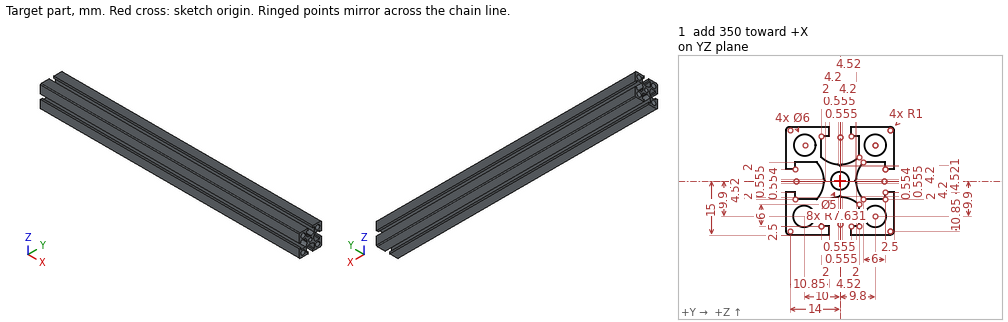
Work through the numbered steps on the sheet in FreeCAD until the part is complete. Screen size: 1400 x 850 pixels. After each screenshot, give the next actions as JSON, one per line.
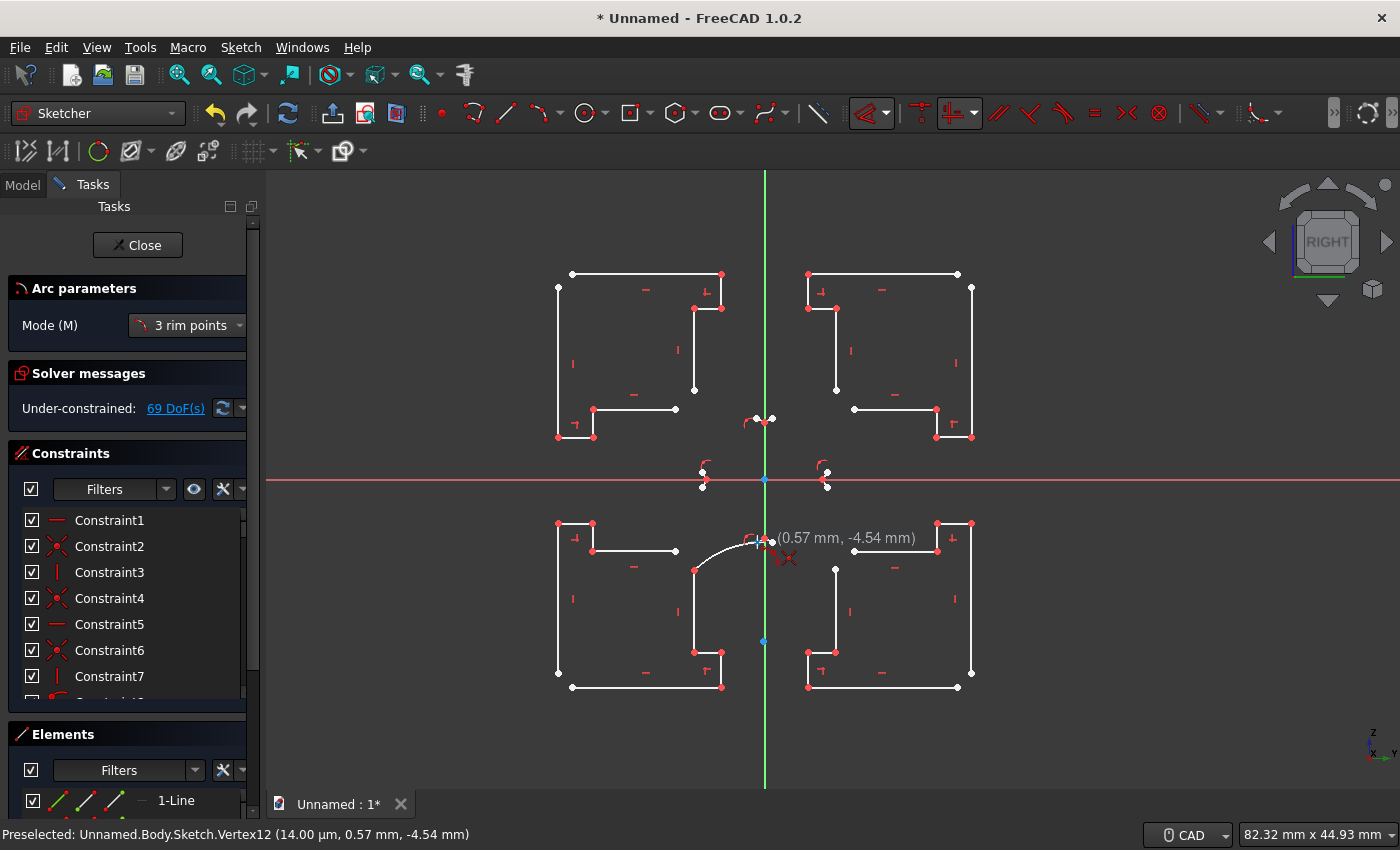
{"action": "left_click", "coordinate": [836, 570]}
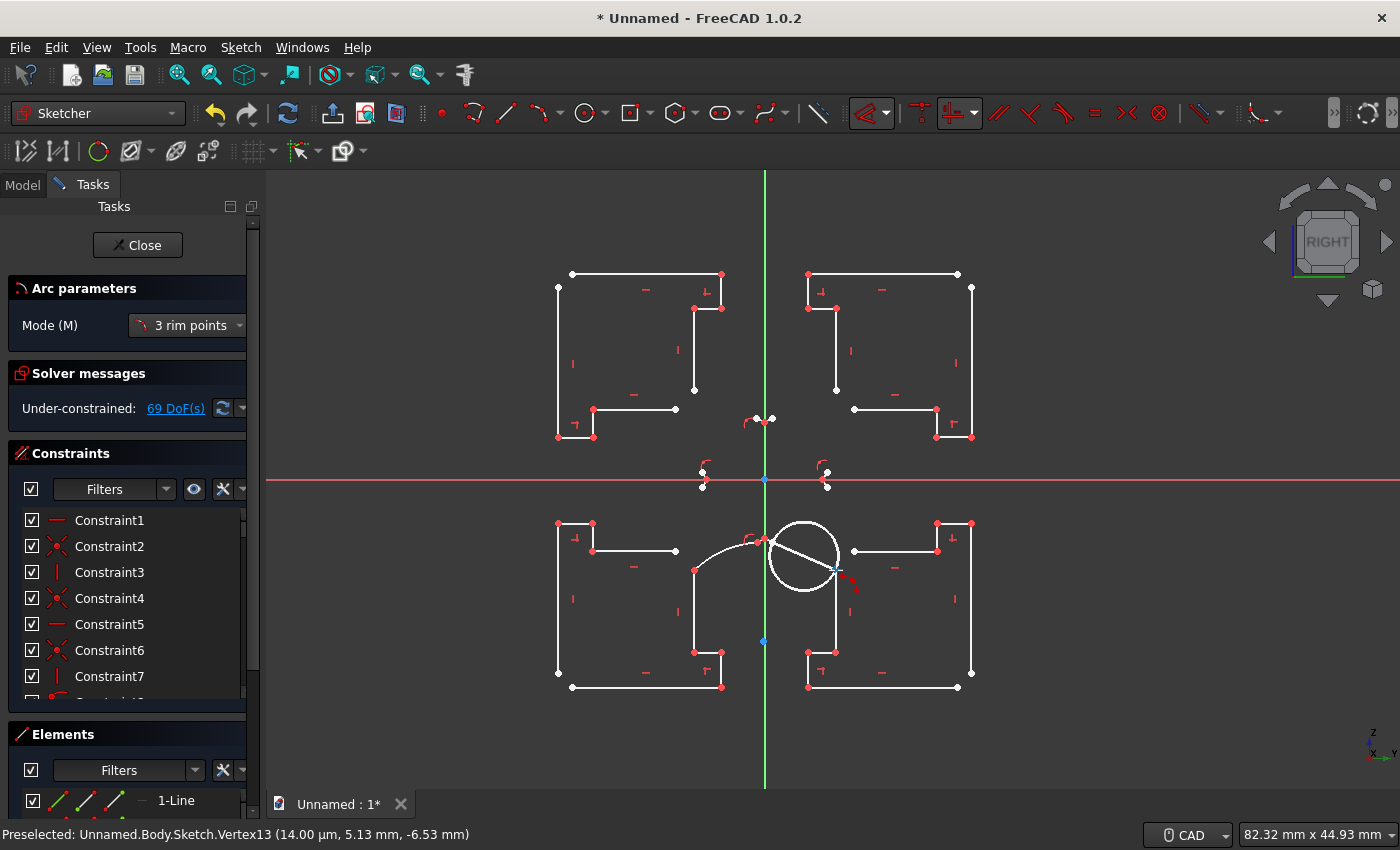
{"action": "scroll", "coordinate": [806, 550], "scroll_direction": "up", "scroll_amount": 6}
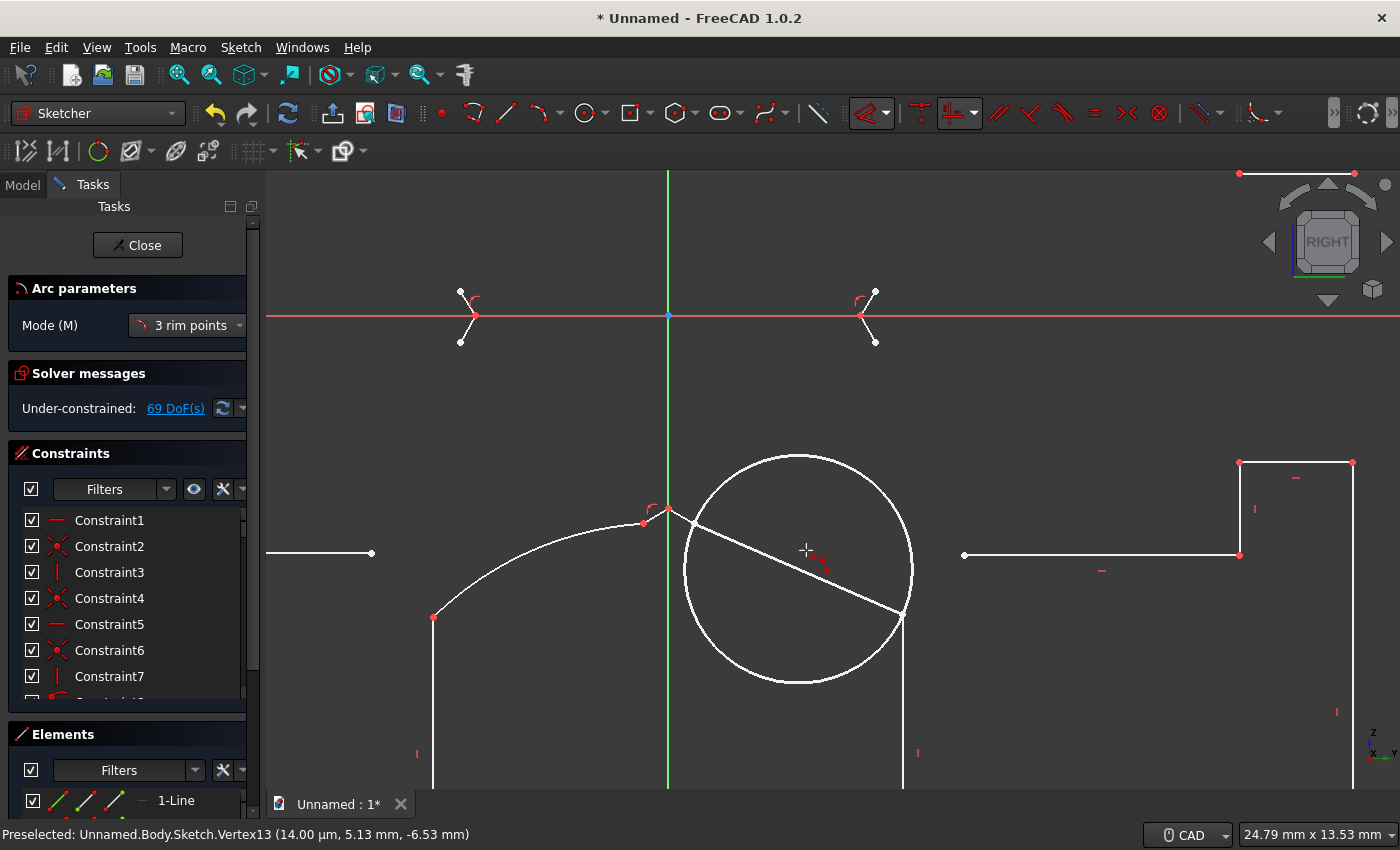
{"action": "left_click", "coordinate": [806, 550]}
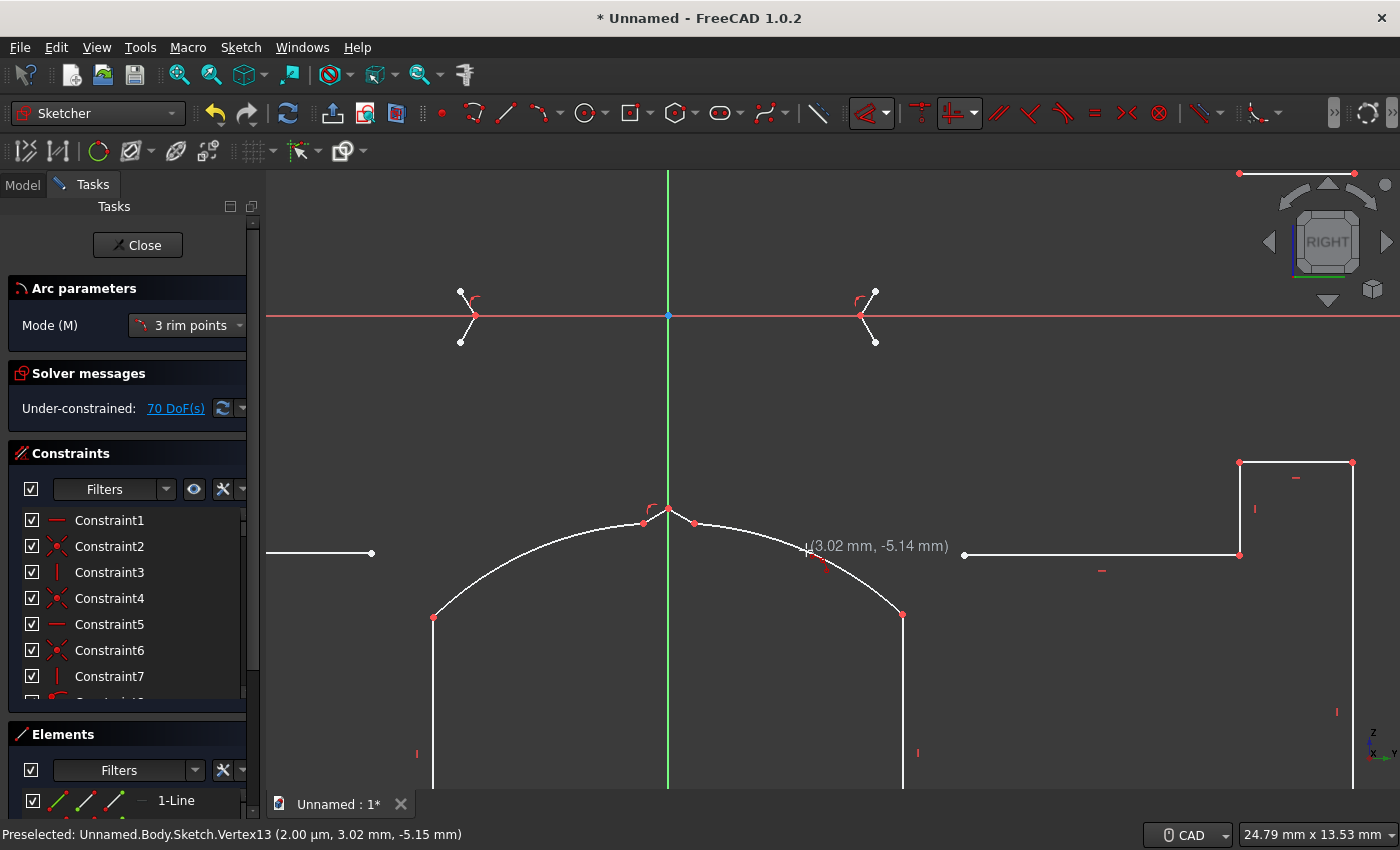
{"action": "scroll", "coordinate": [806, 550], "scroll_direction": "down", "scroll_amount": 6}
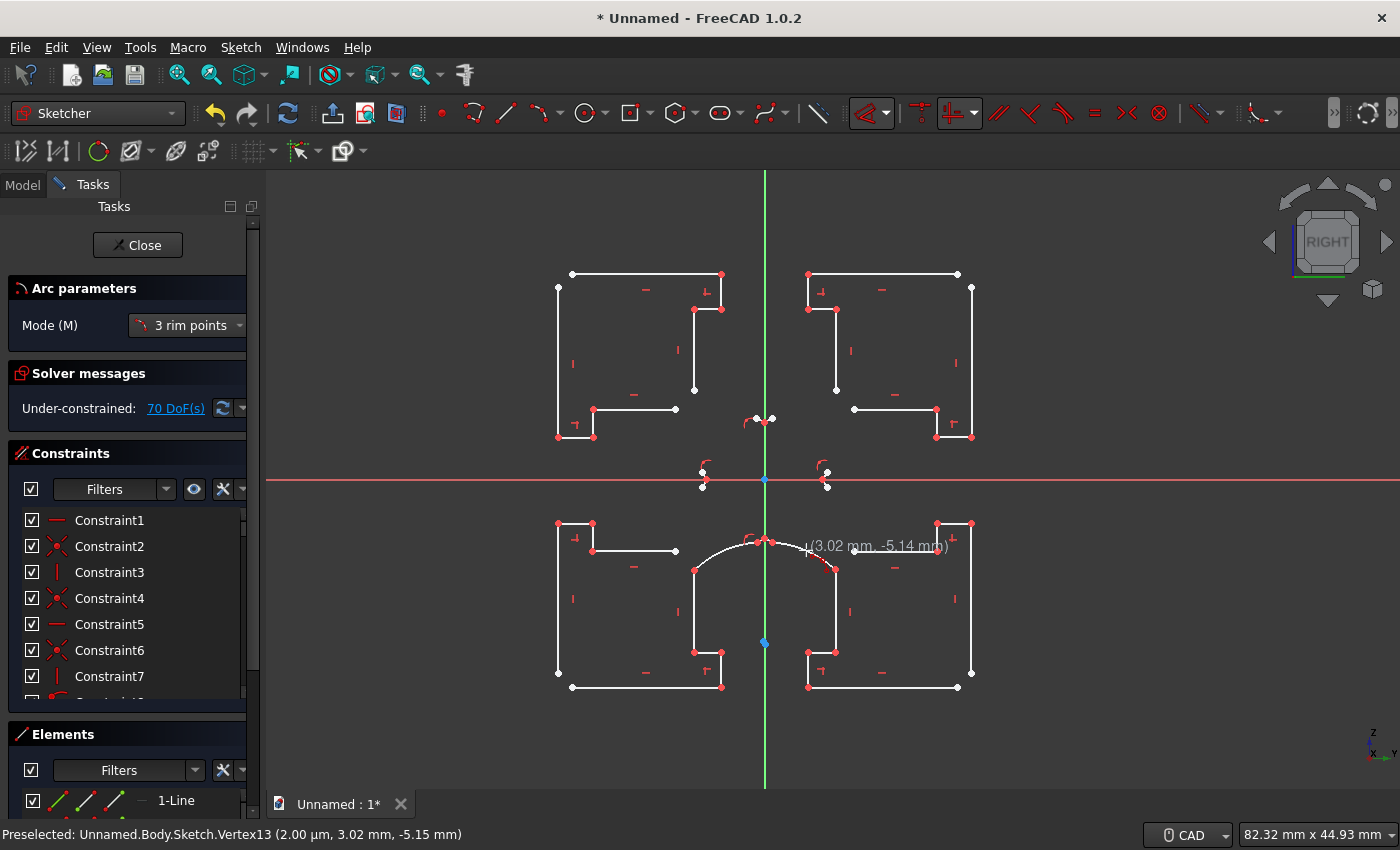
{"action": "left_click", "coordinate": [958, 688]}
{"action": "left_click", "coordinate": [971, 674]}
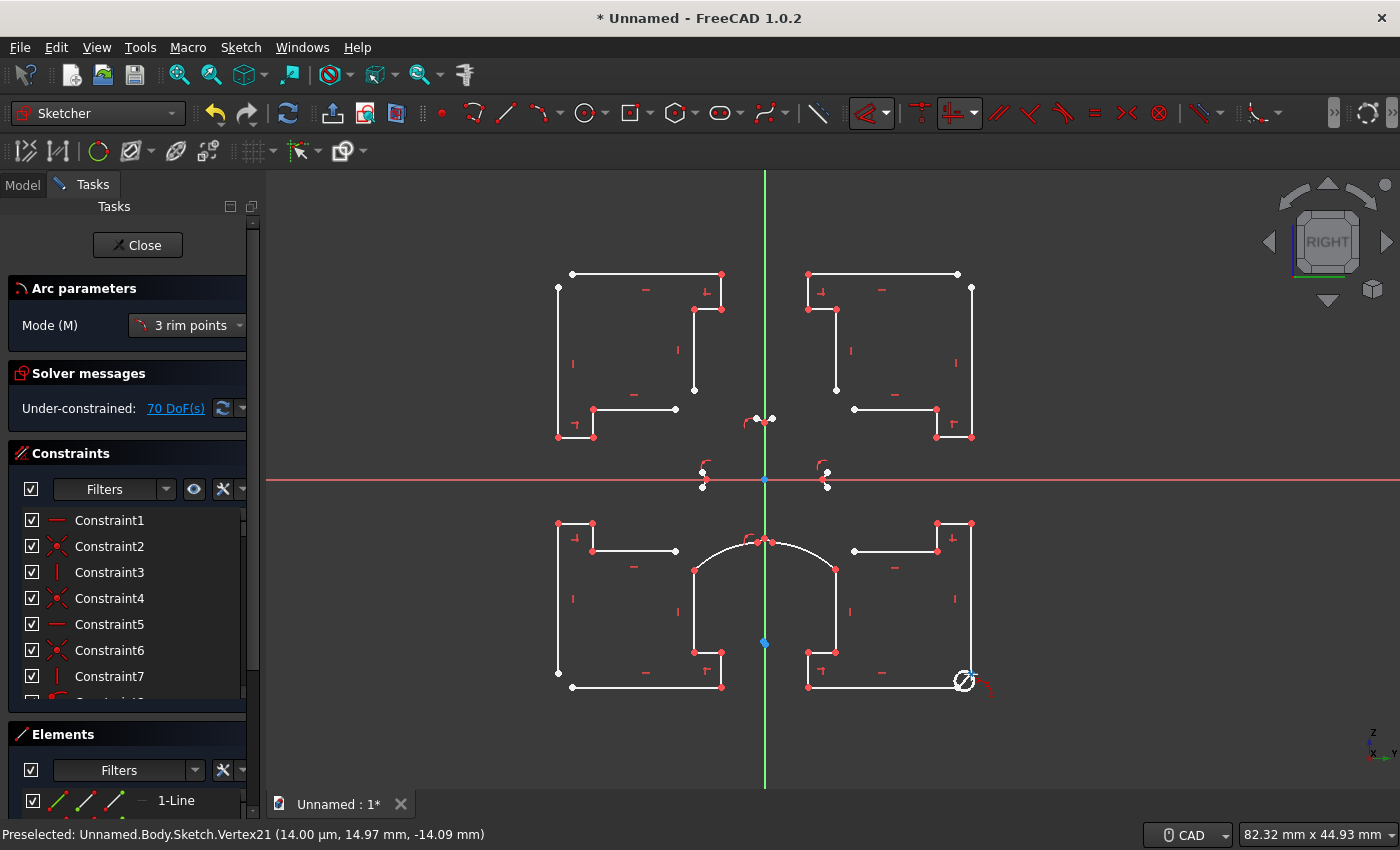
{"action": "scroll", "coordinate": [967, 683], "scroll_direction": "up", "scroll_amount": 7}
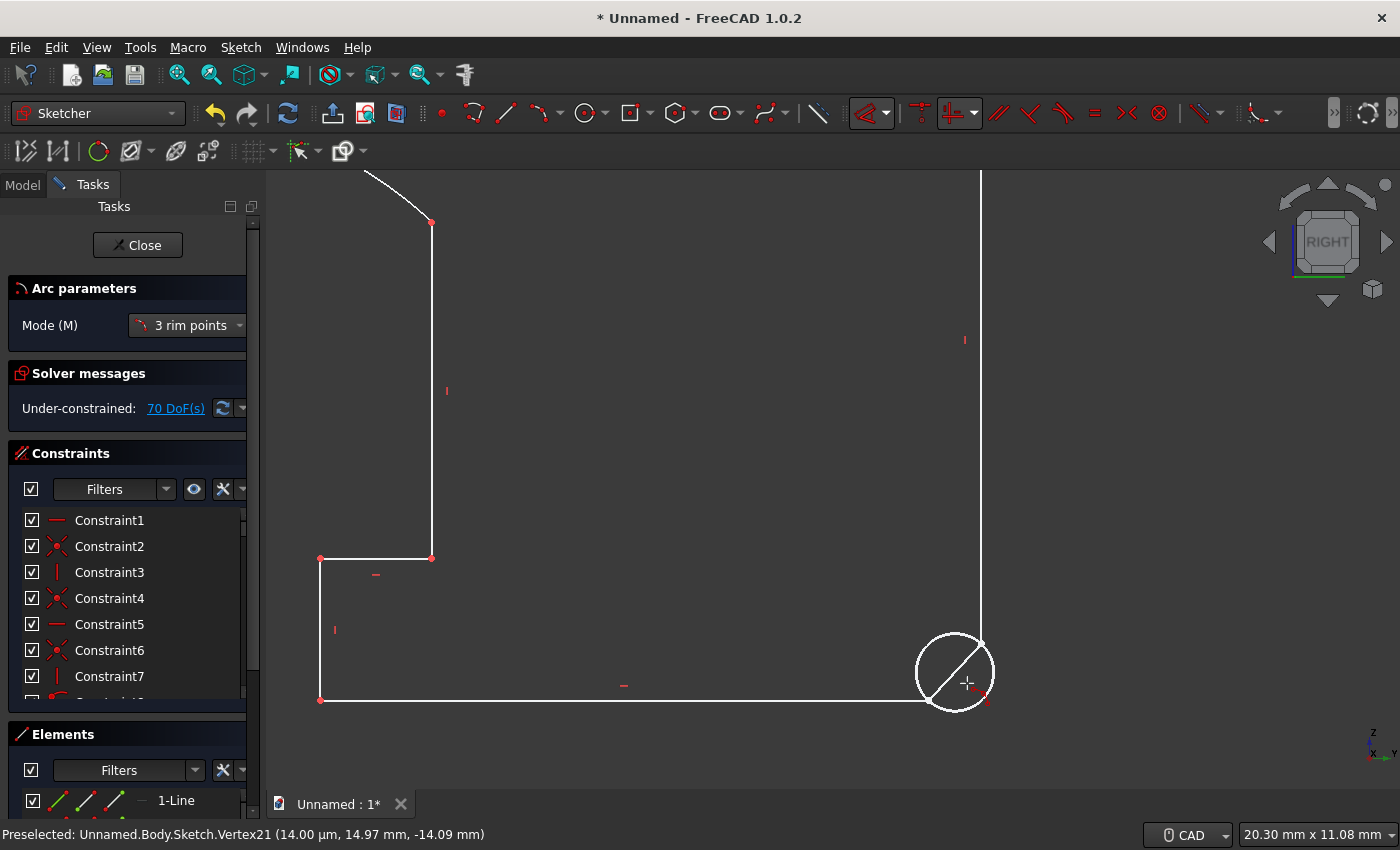
{"action": "left_click", "coordinate": [967, 679]}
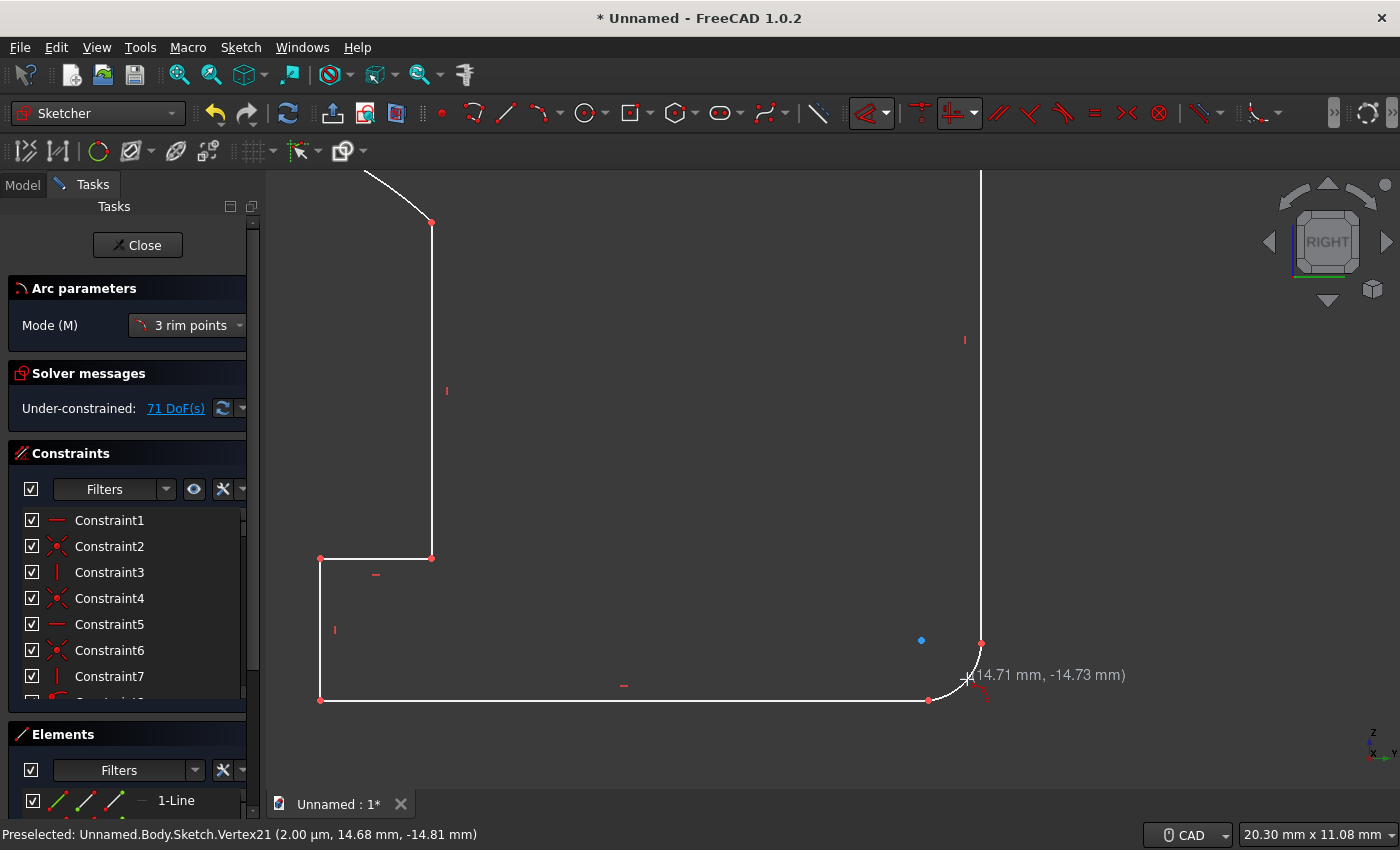
{"action": "scroll", "coordinate": [967, 683], "scroll_direction": "down", "scroll_amount": 7}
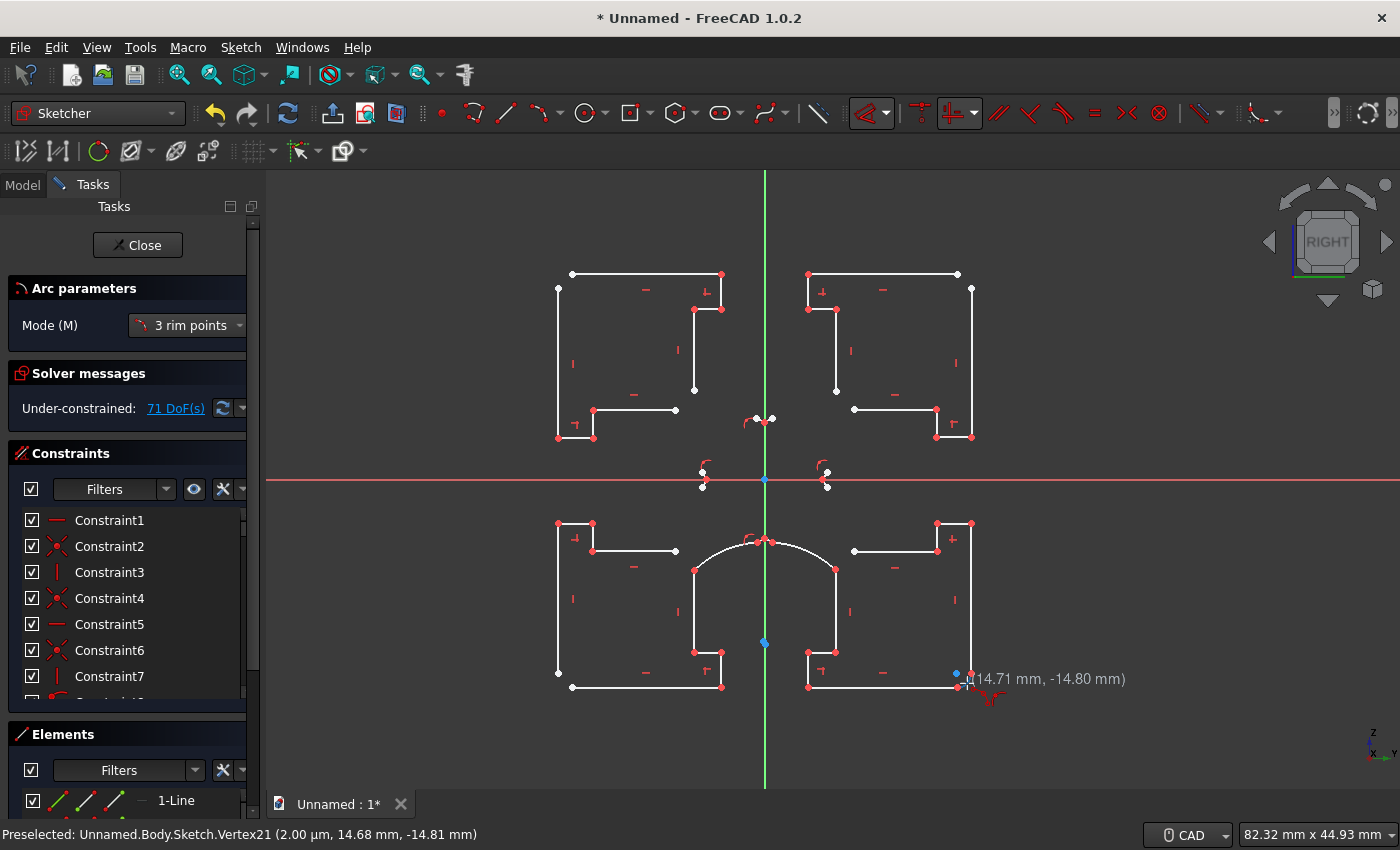
{"action": "left_click", "coordinate": [854, 552]}